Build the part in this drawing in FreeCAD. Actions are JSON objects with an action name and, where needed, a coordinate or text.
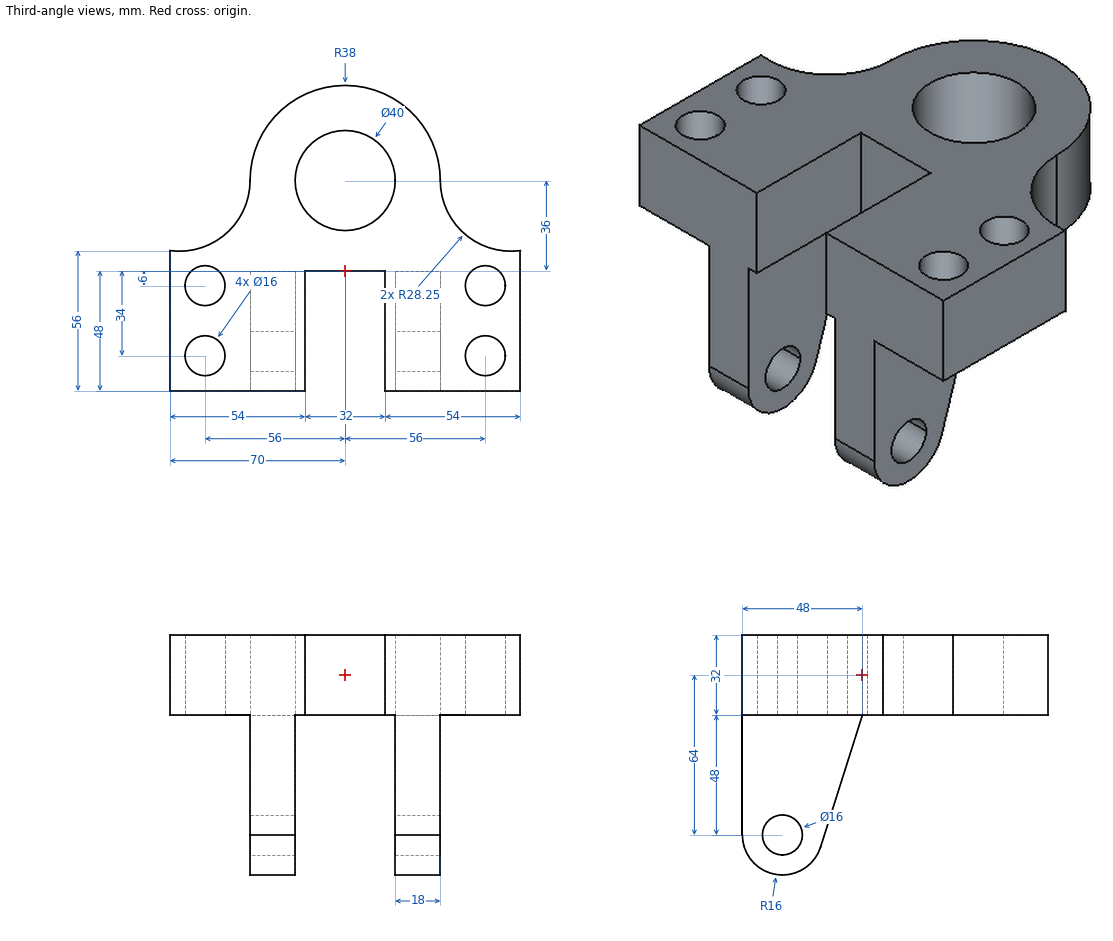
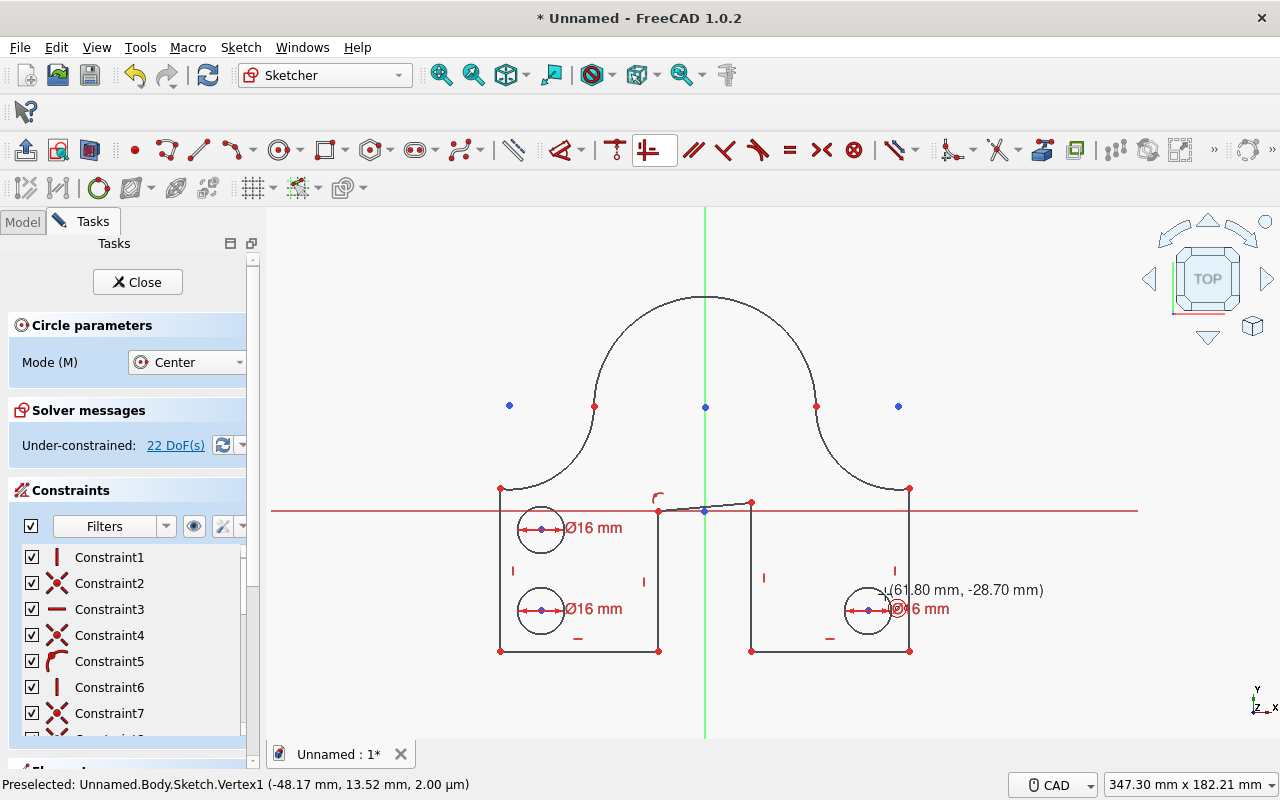
{"action": "left_click", "coordinate": [868, 529]}
{"action": "mouse_move", "coordinate": [885, 545]}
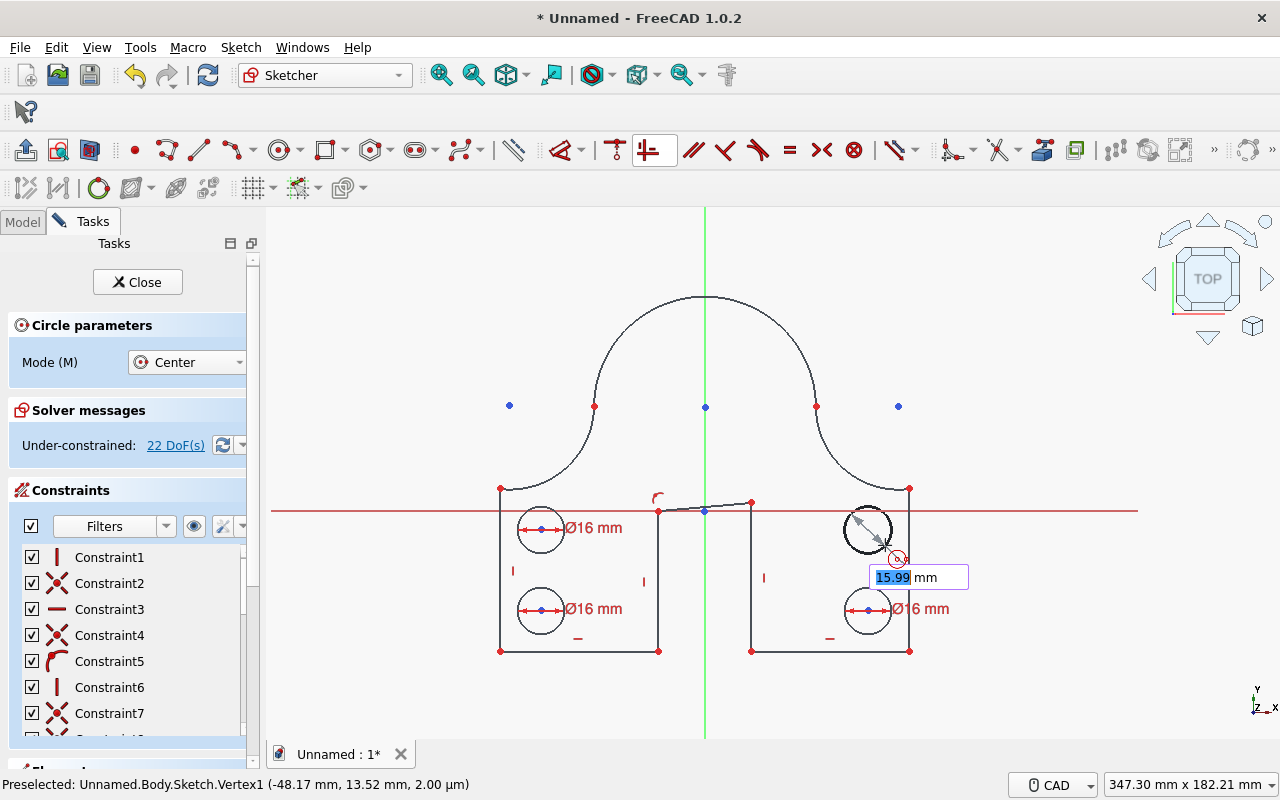
{"action": "type", "text": "16"}
{"action": "key", "text": "Return"}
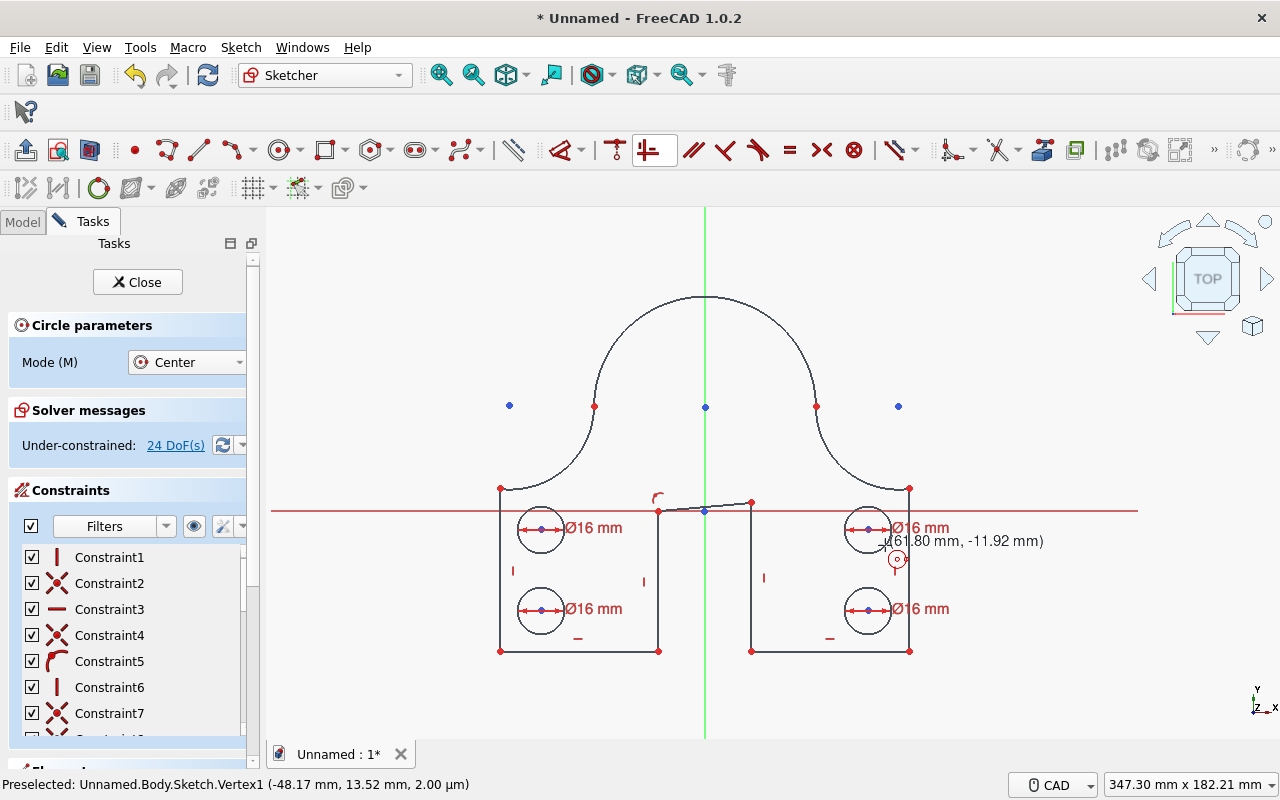
{"action": "left_click", "coordinate": [705, 406]}
{"action": "mouse_move", "coordinate": [746, 365]}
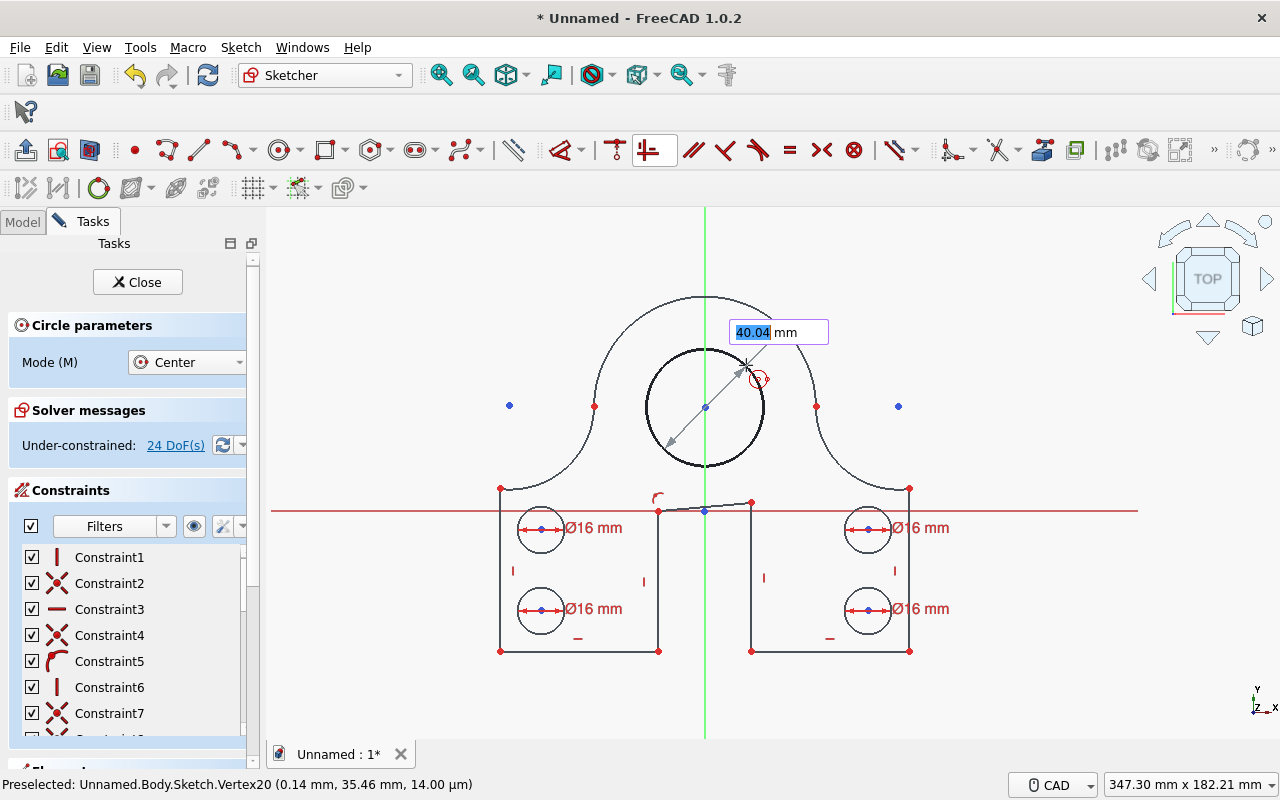
{"action": "type", "text": "40"}
{"action": "key", "text": "Return"}
{"action": "key", "text": "Escape"}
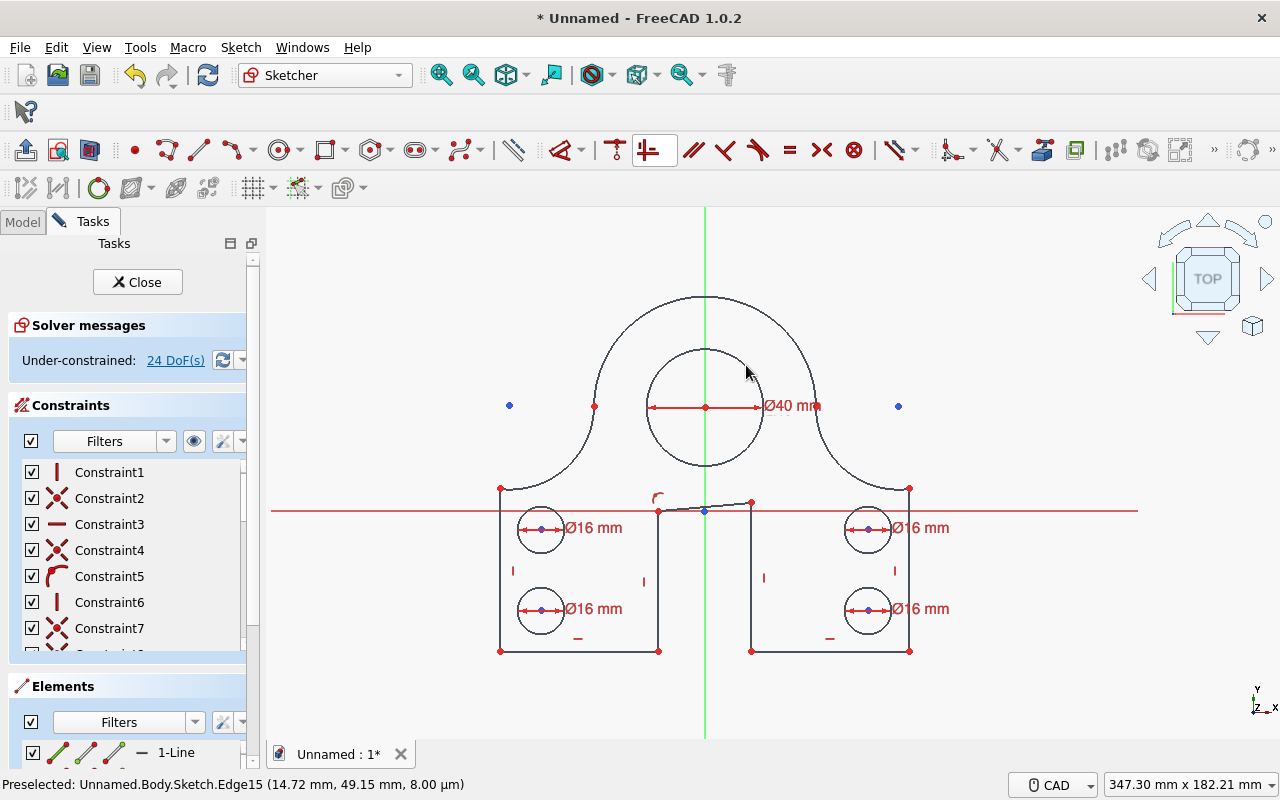
{"action": "left_click", "coordinate": [826, 447]}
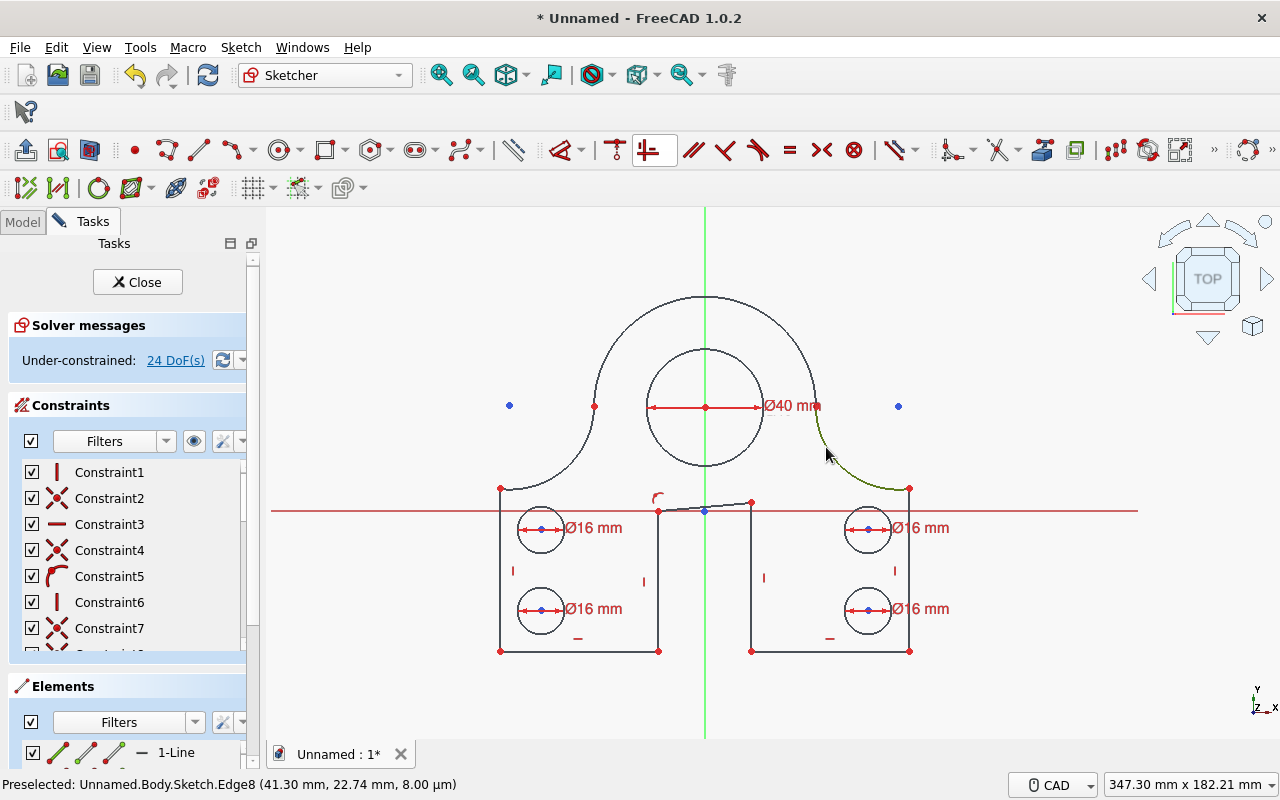
{"action": "left_click", "coordinate": [770, 318]}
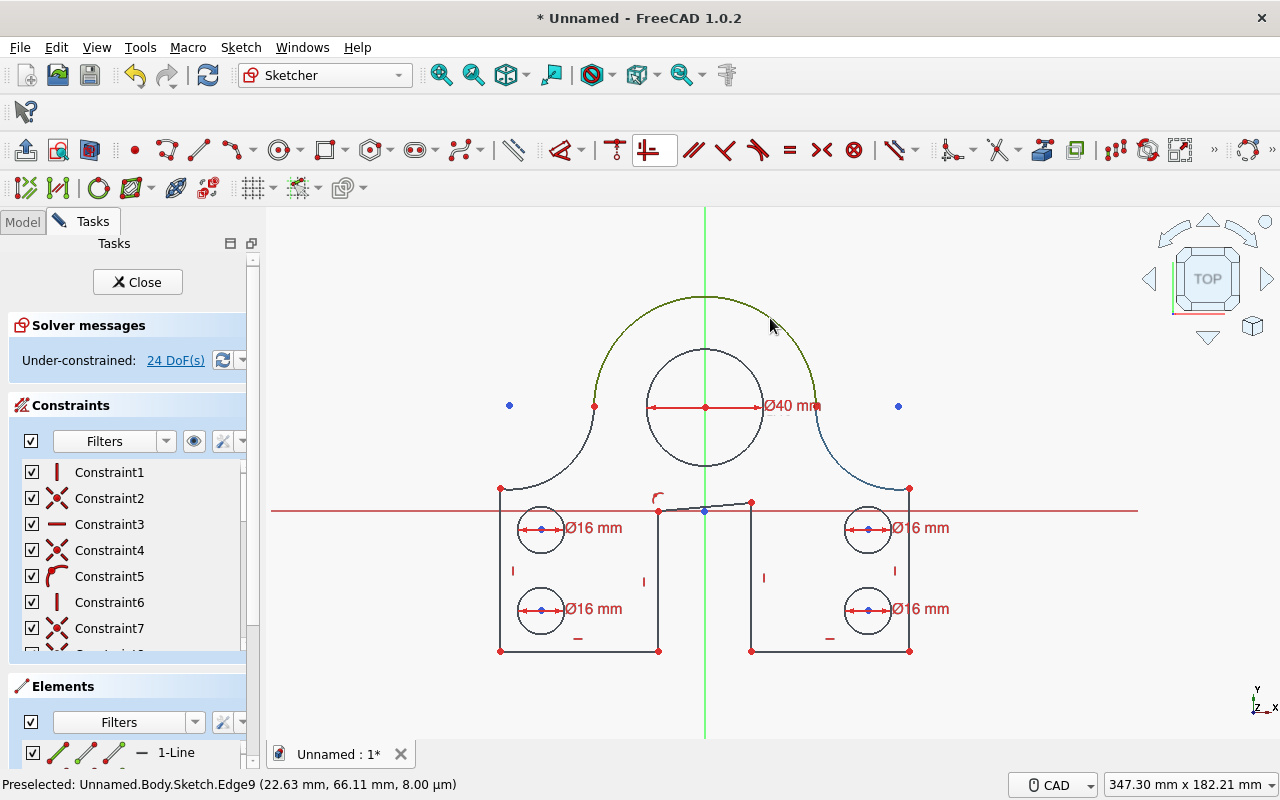
{"action": "left_click", "coordinate": [758, 150]}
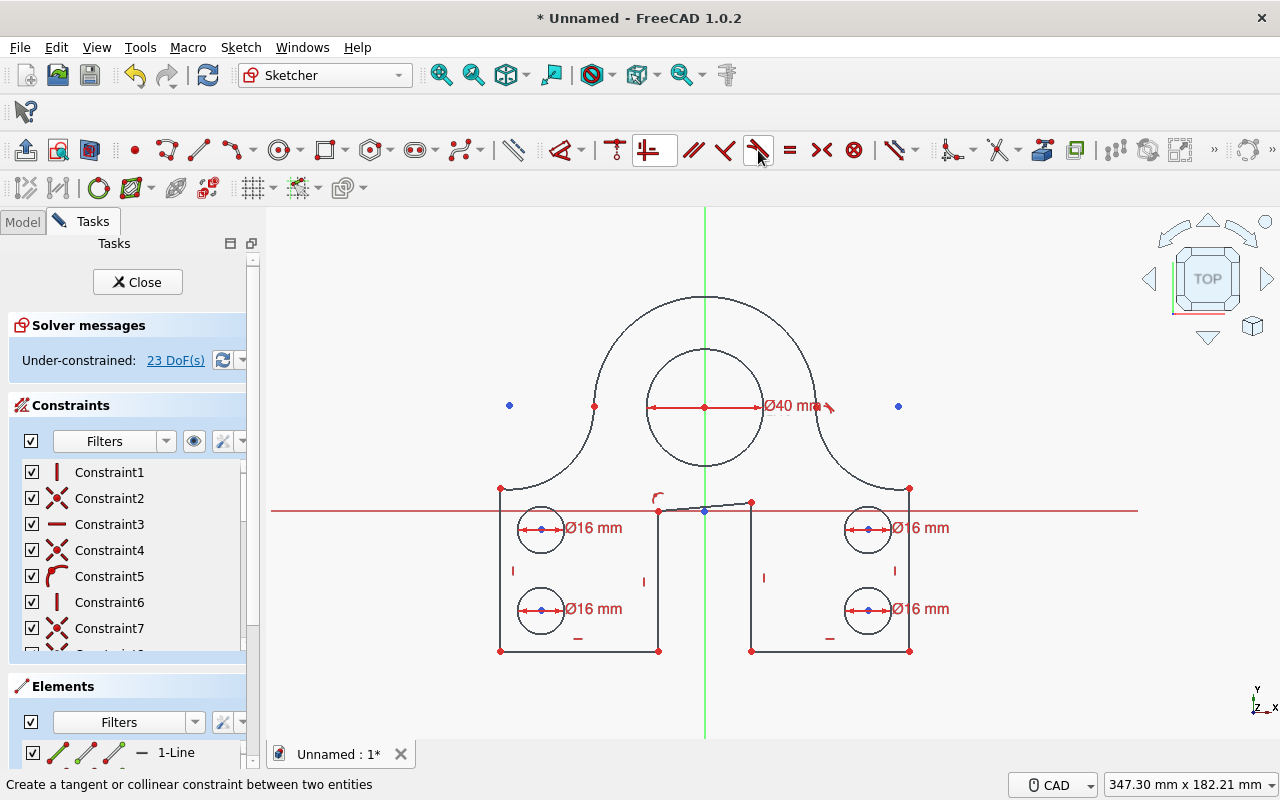
{"action": "left_click", "coordinate": [770, 318]}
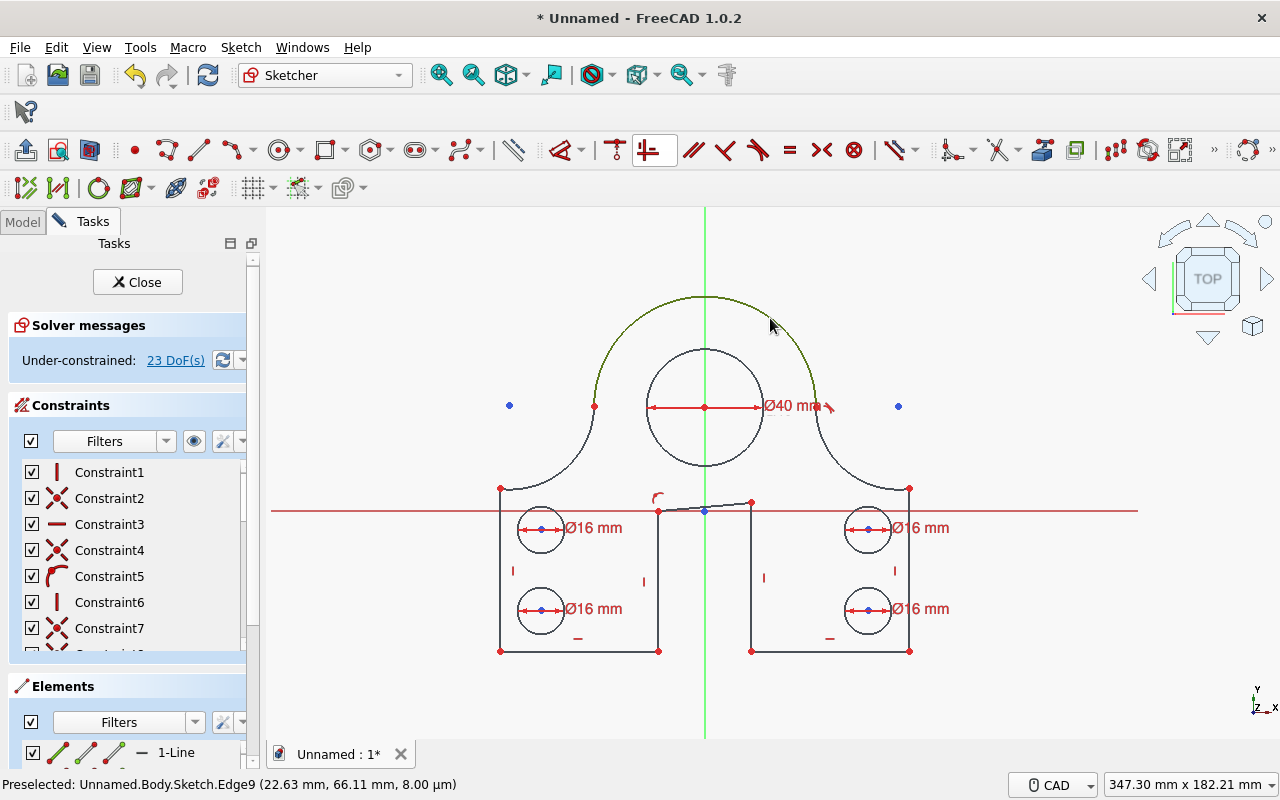
{"action": "left_click", "coordinate": [541, 483]}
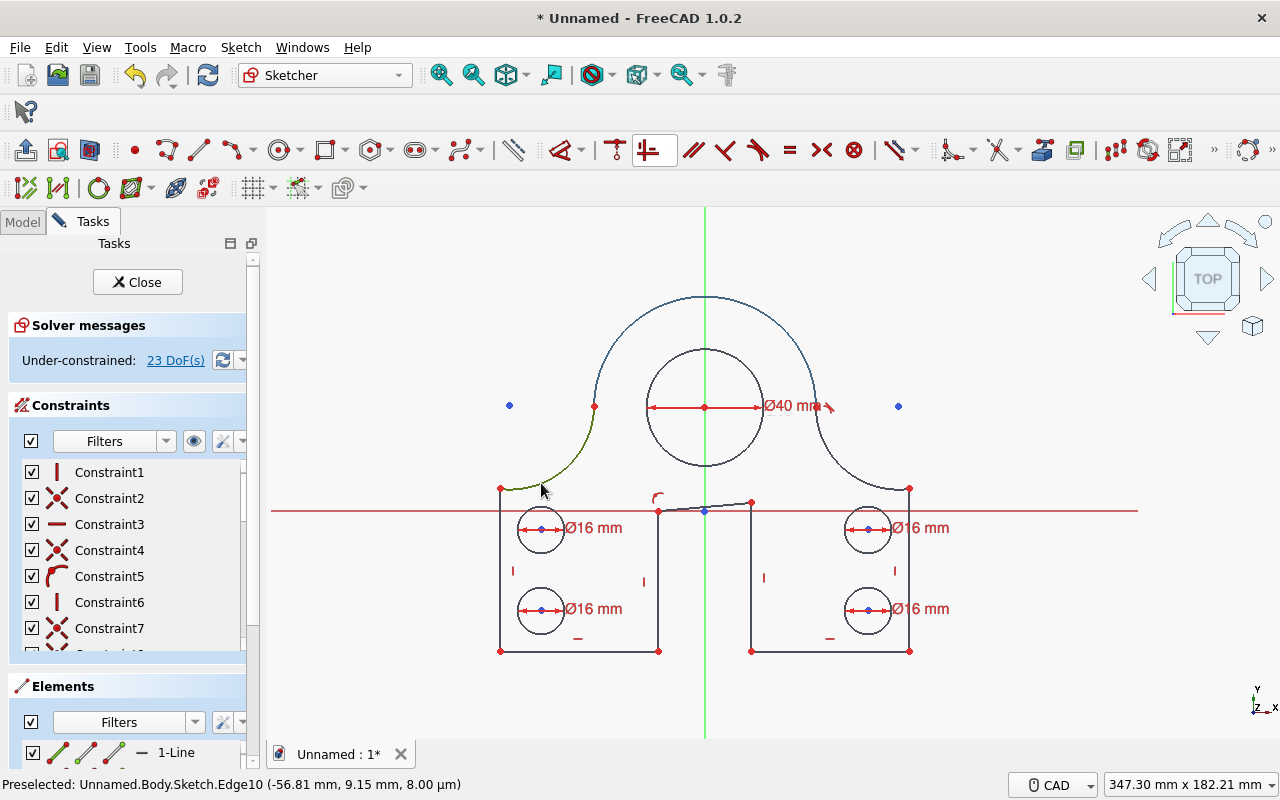
{"action": "left_click", "coordinate": [758, 150]}